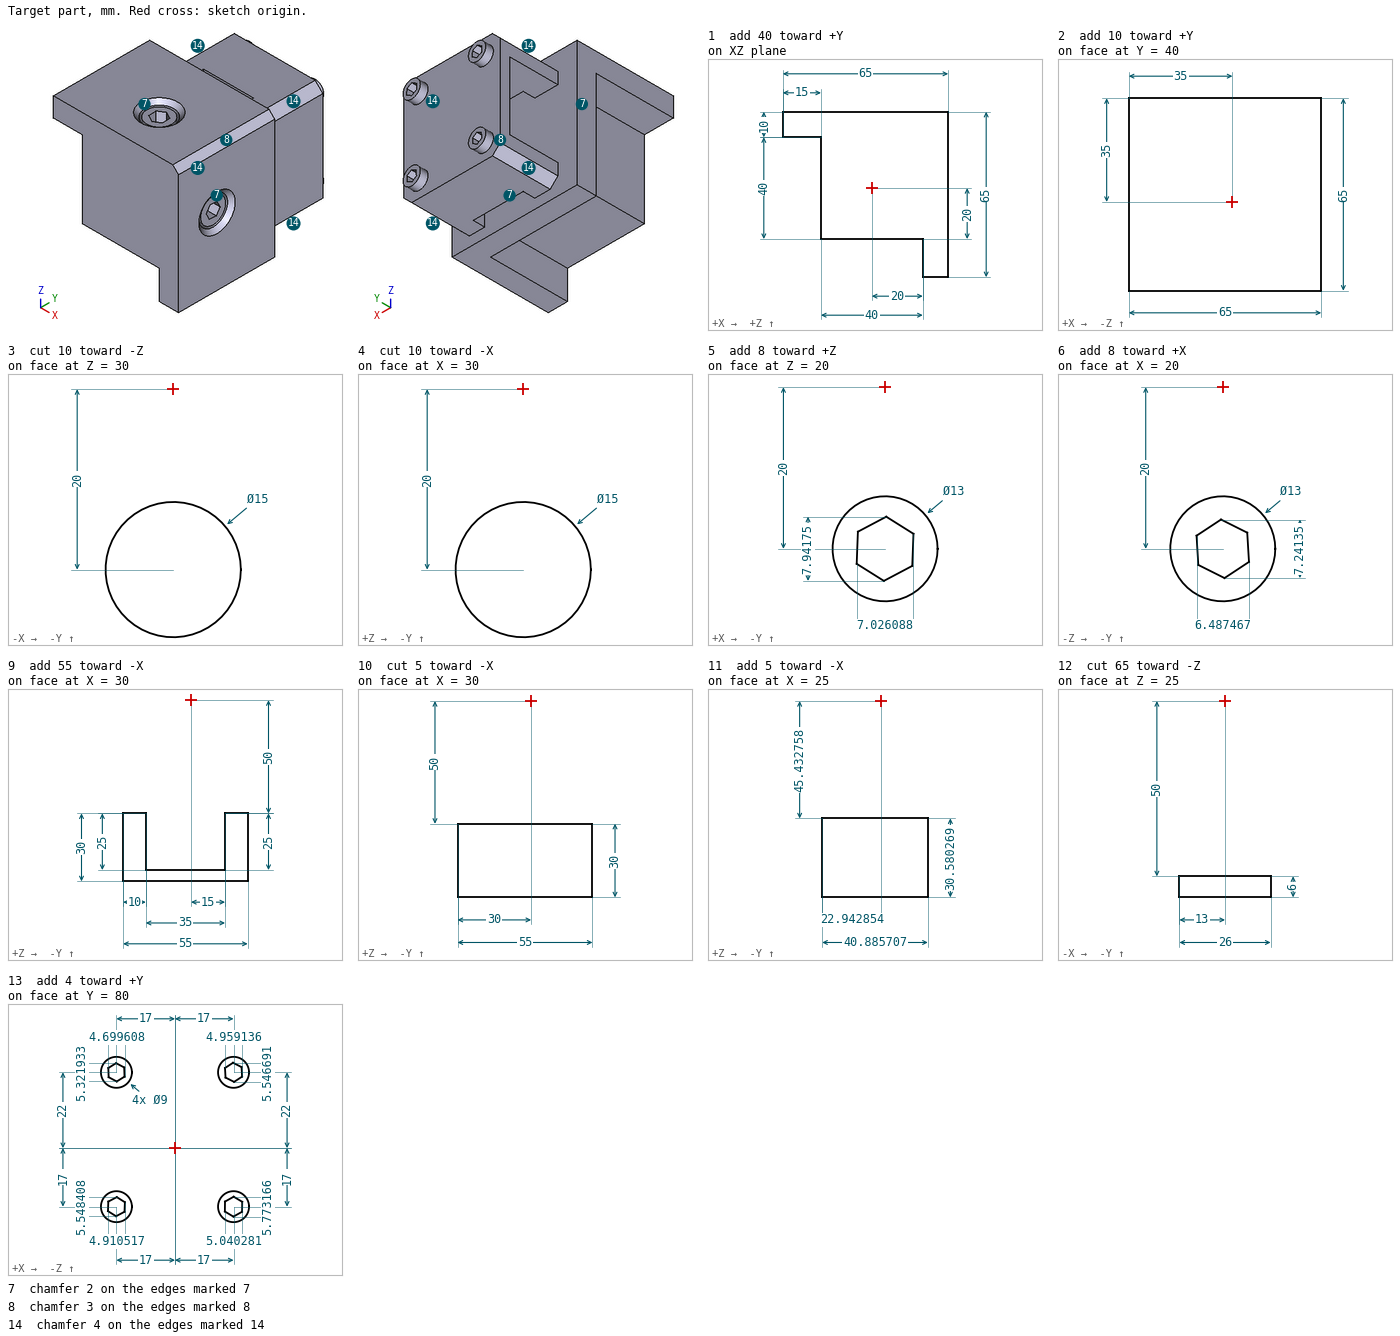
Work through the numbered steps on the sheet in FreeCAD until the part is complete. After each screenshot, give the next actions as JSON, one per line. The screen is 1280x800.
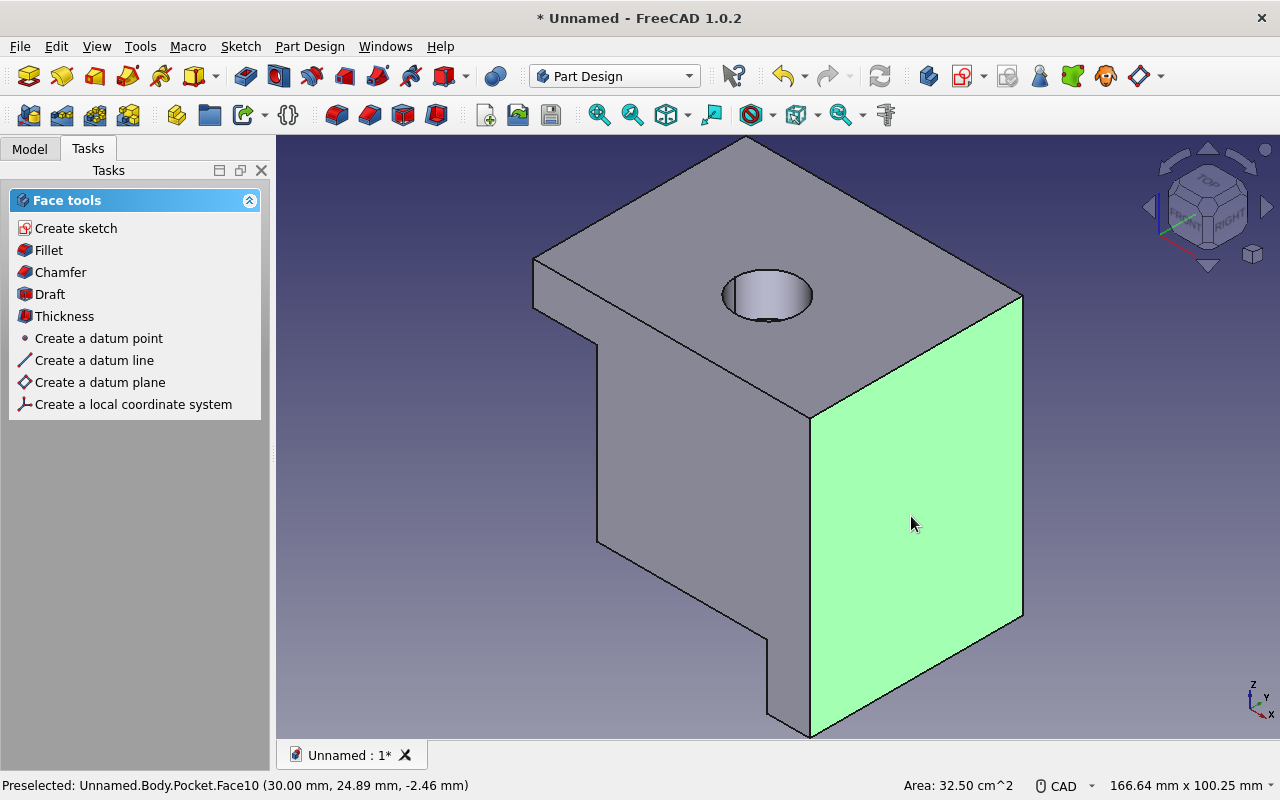
{"action": "left_click", "coordinate": [962, 76]}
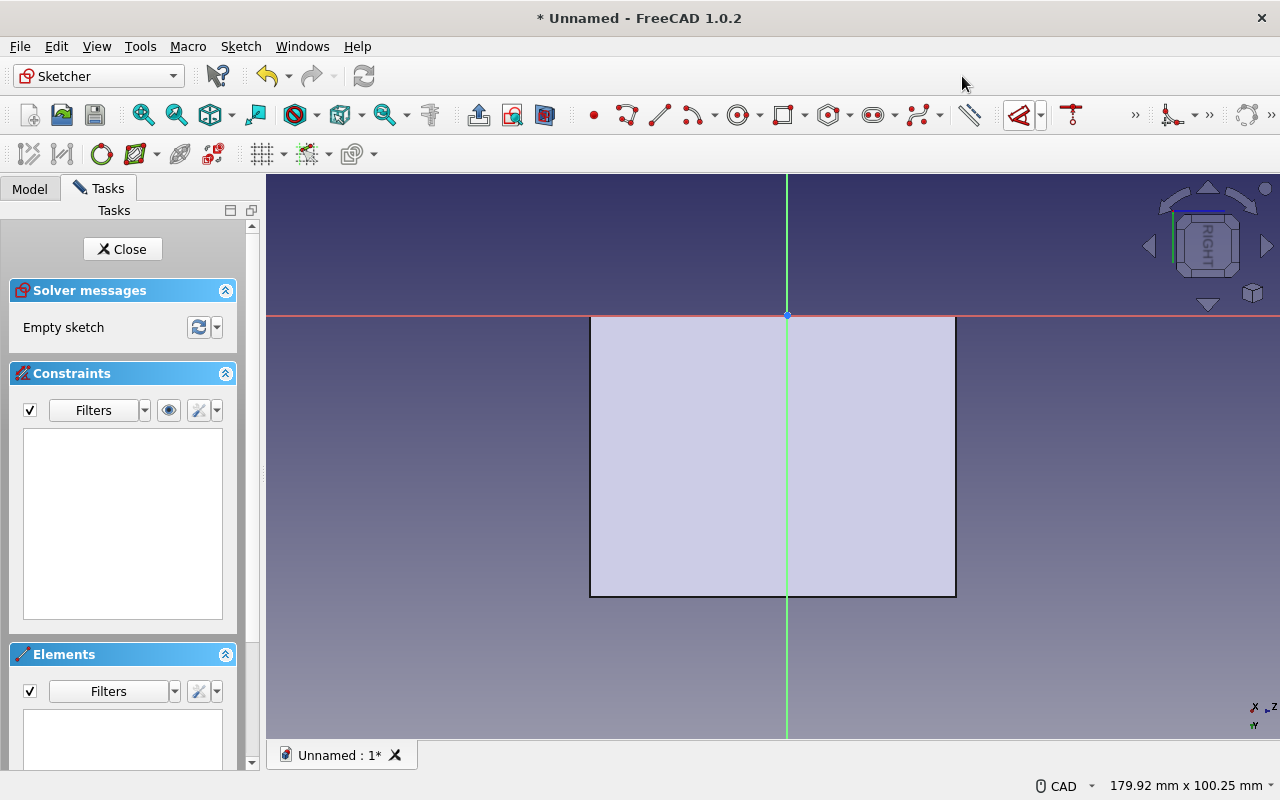
{"action": "scroll", "coordinate": [854, 341], "scroll_direction": "up", "scroll_amount": 4}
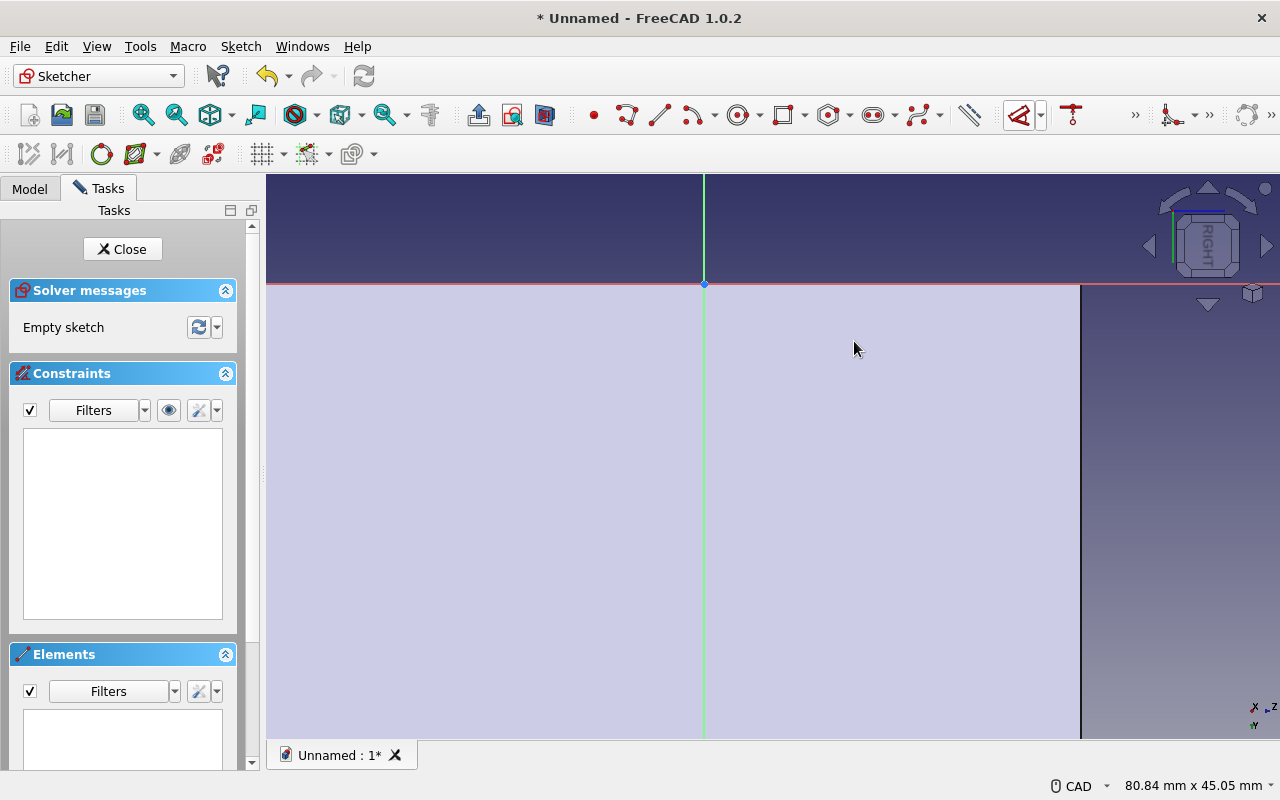
{"action": "left_click", "coordinate": [738, 116]}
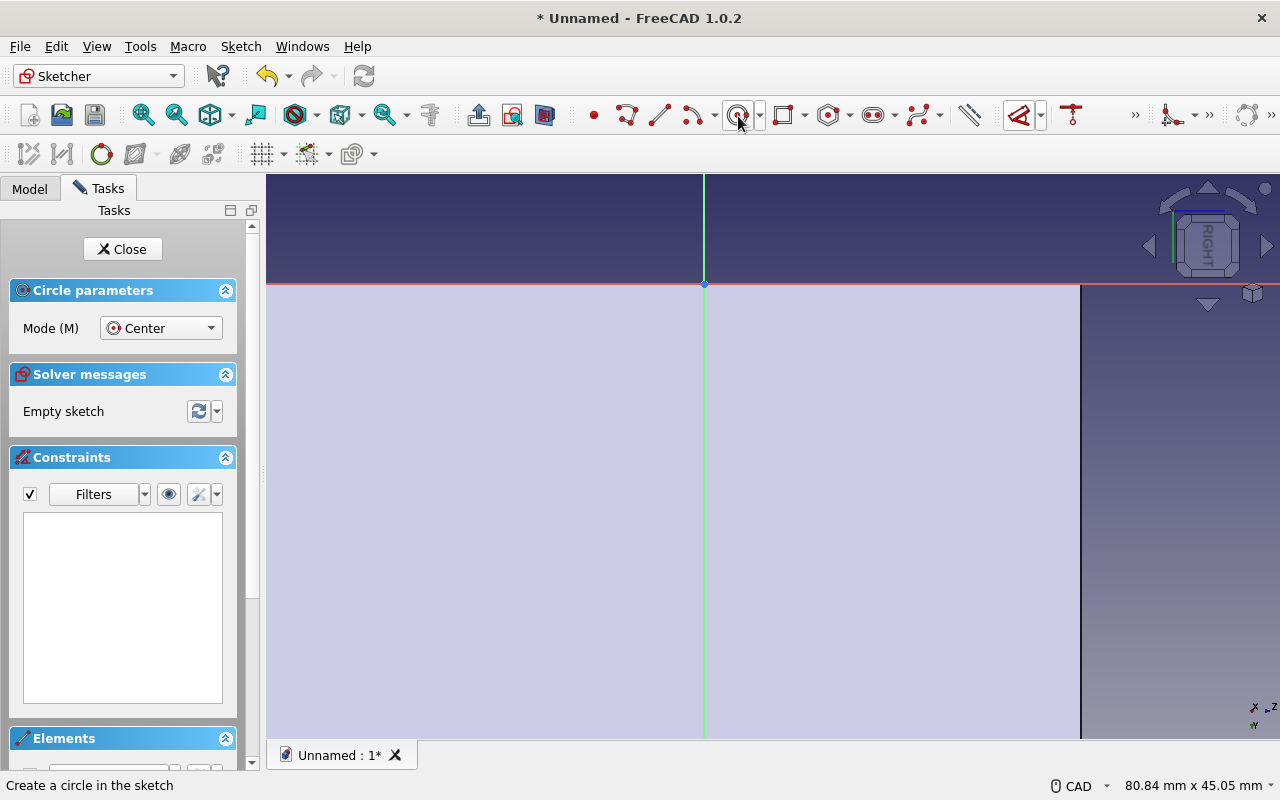
{"action": "left_click", "coordinate": [704, 535]}
{"action": "mouse_move", "coordinate": [771, 468]}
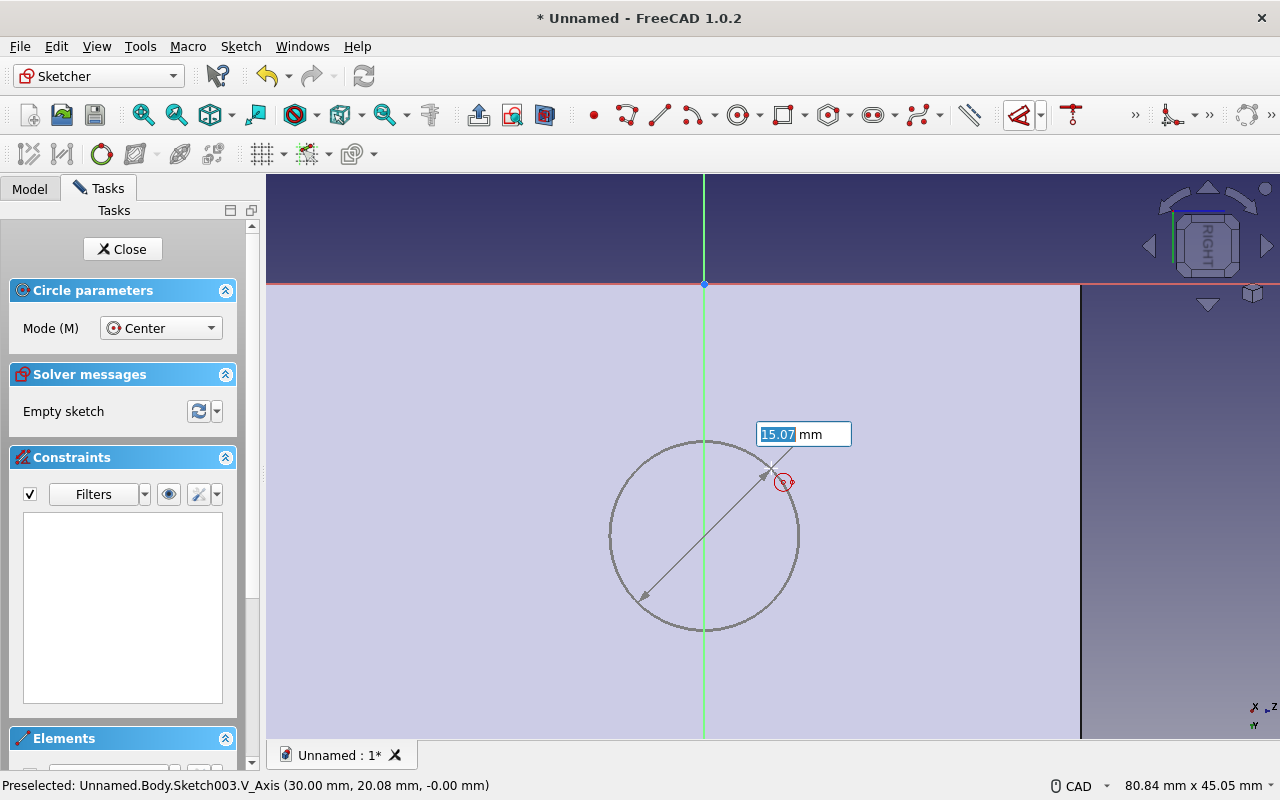
{"action": "type", "text": "15"}
{"action": "key", "text": "Return"}
{"action": "key", "text": "Escape"}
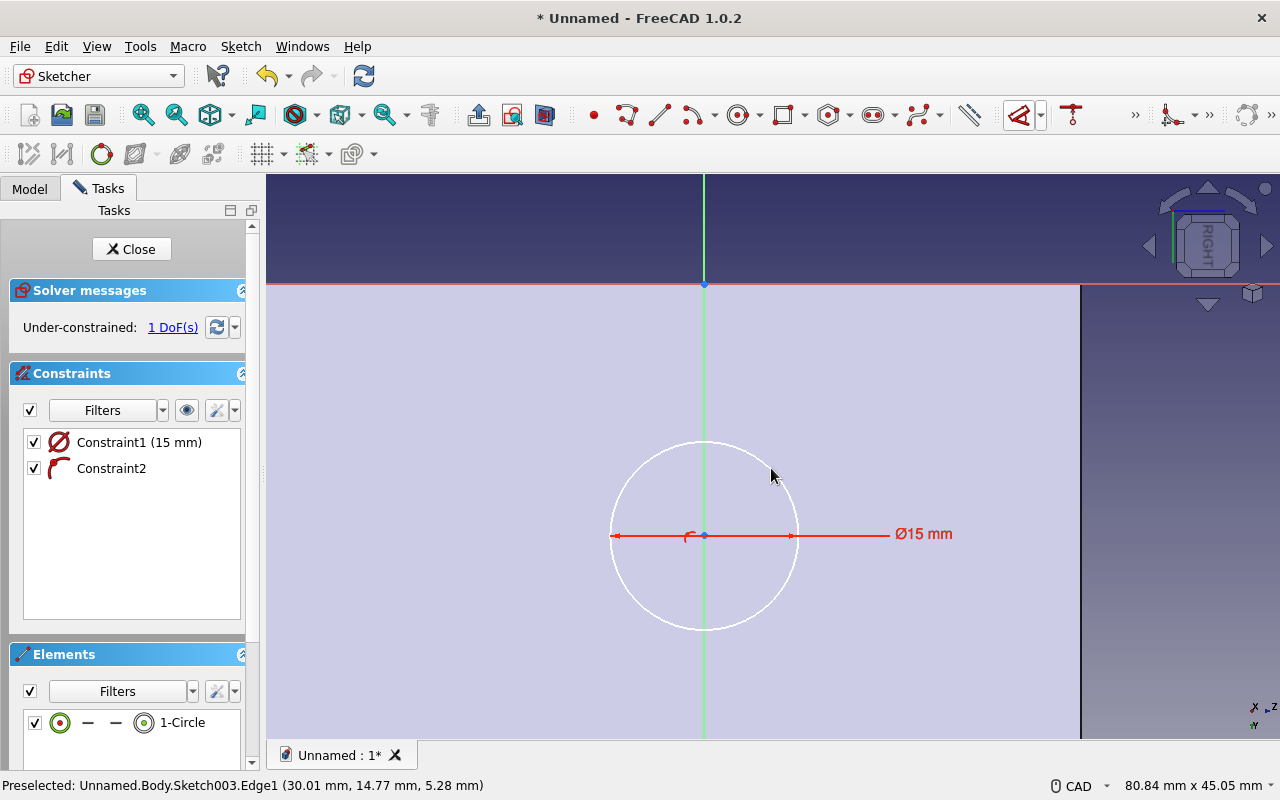
{"action": "left_click", "coordinate": [704, 536]}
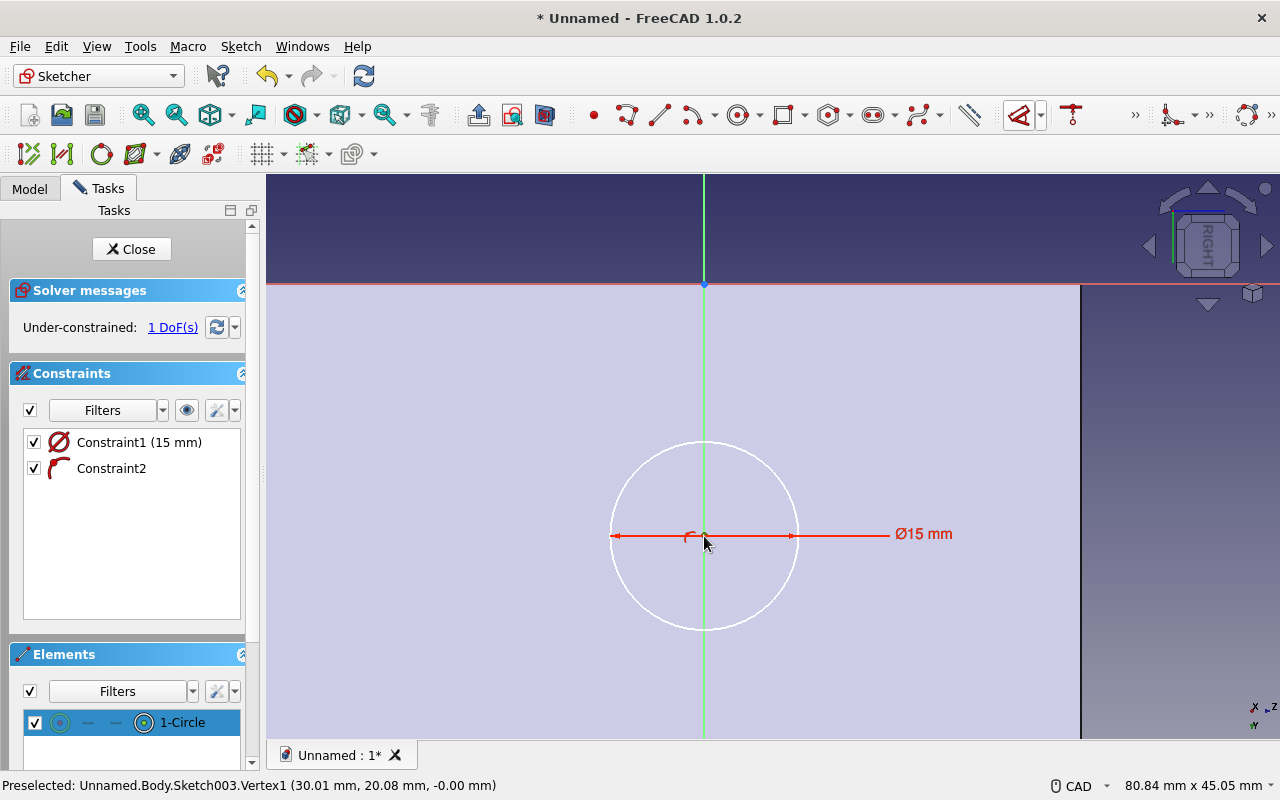
{"action": "left_click", "coordinate": [1040, 116]}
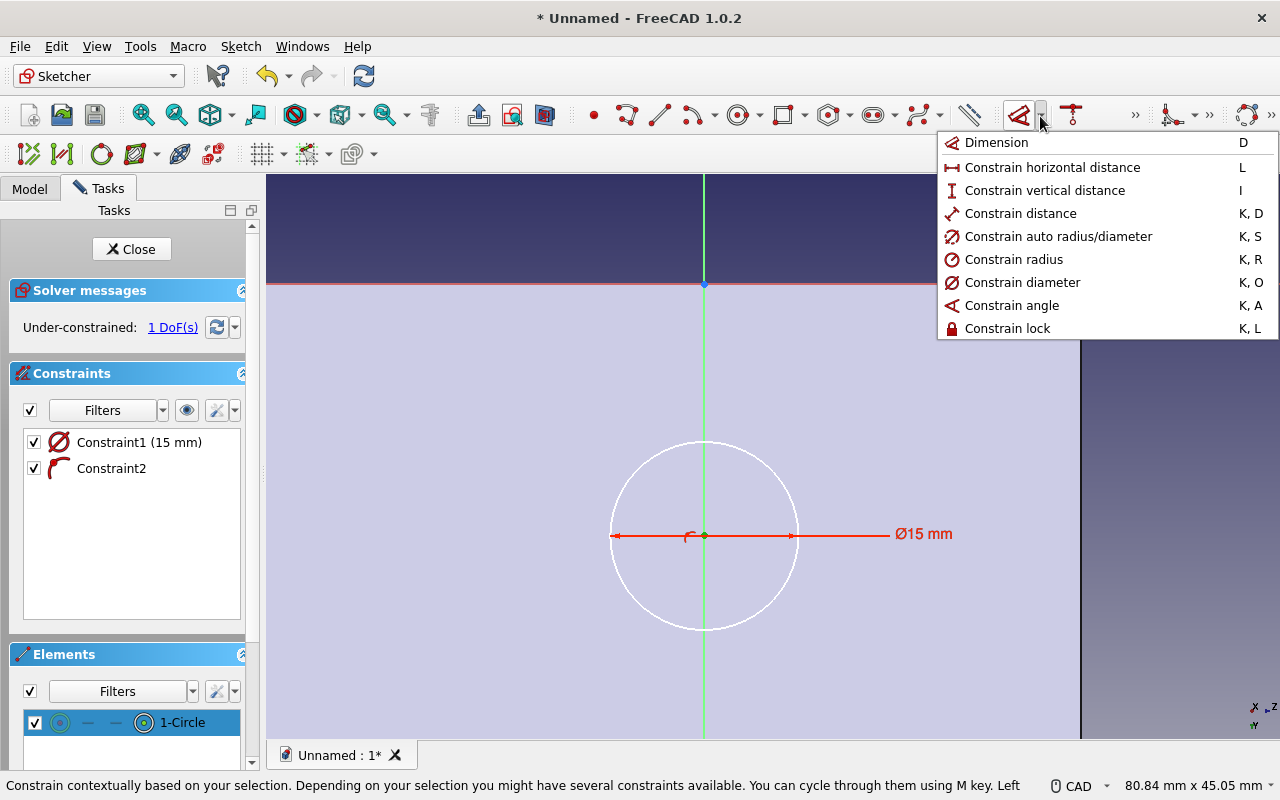
{"action": "left_click", "coordinate": [1108, 190]}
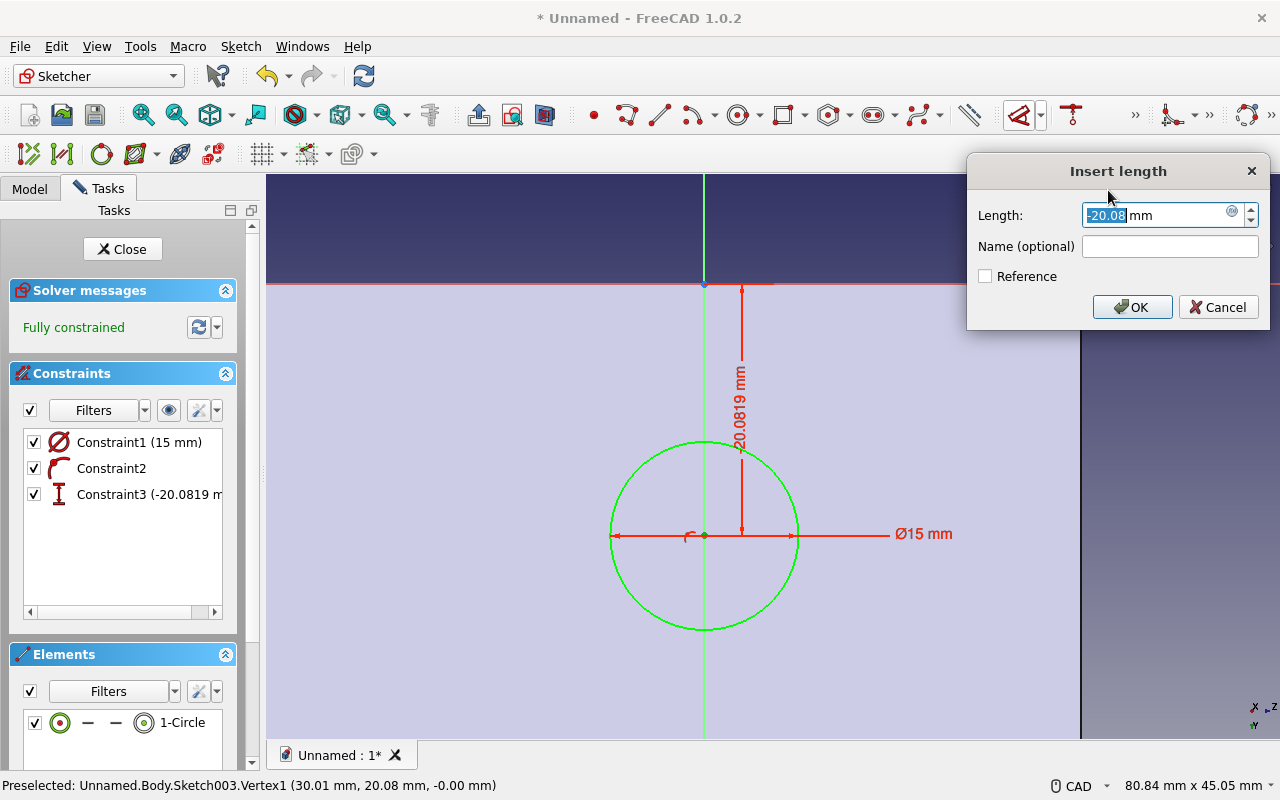
{"action": "type", "text": "-20"}
{"action": "key", "text": "Return"}